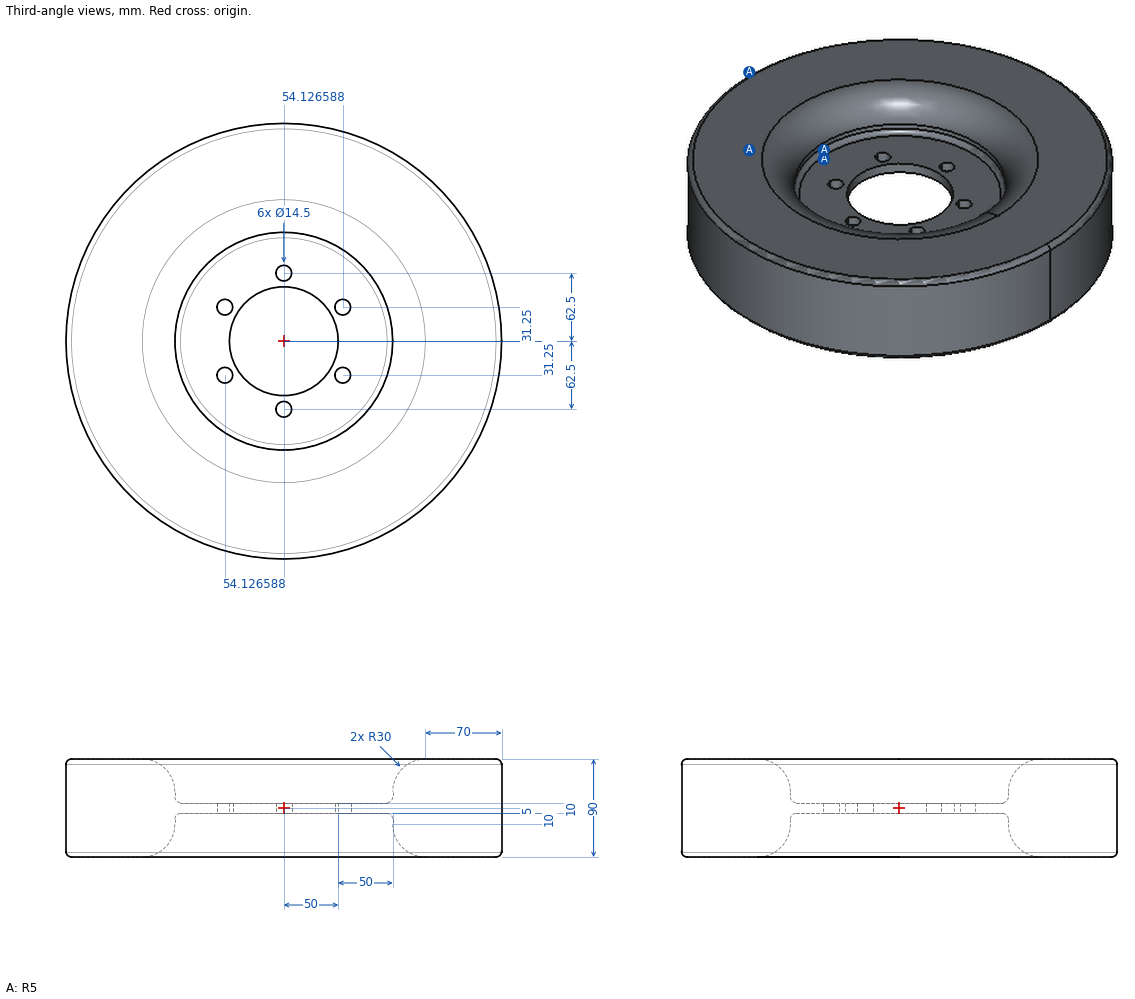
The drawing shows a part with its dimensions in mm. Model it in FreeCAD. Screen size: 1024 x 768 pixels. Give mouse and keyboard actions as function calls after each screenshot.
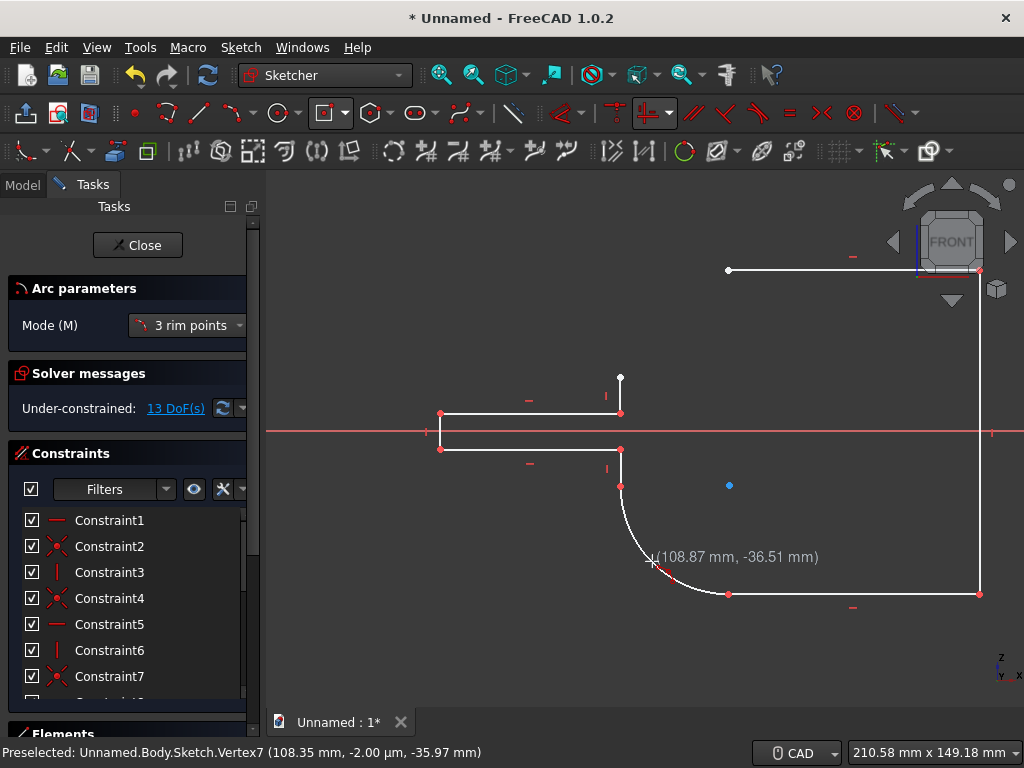
click(620, 378)
click(728, 270)
click(652, 300)
key(Escape)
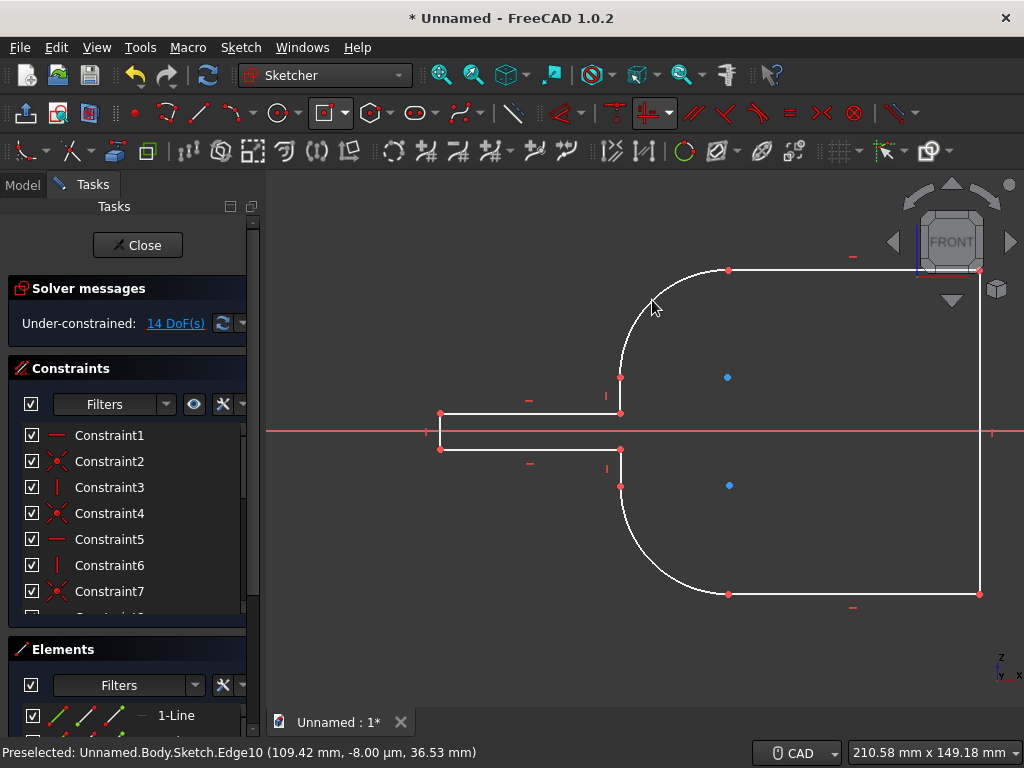
click(804, 270)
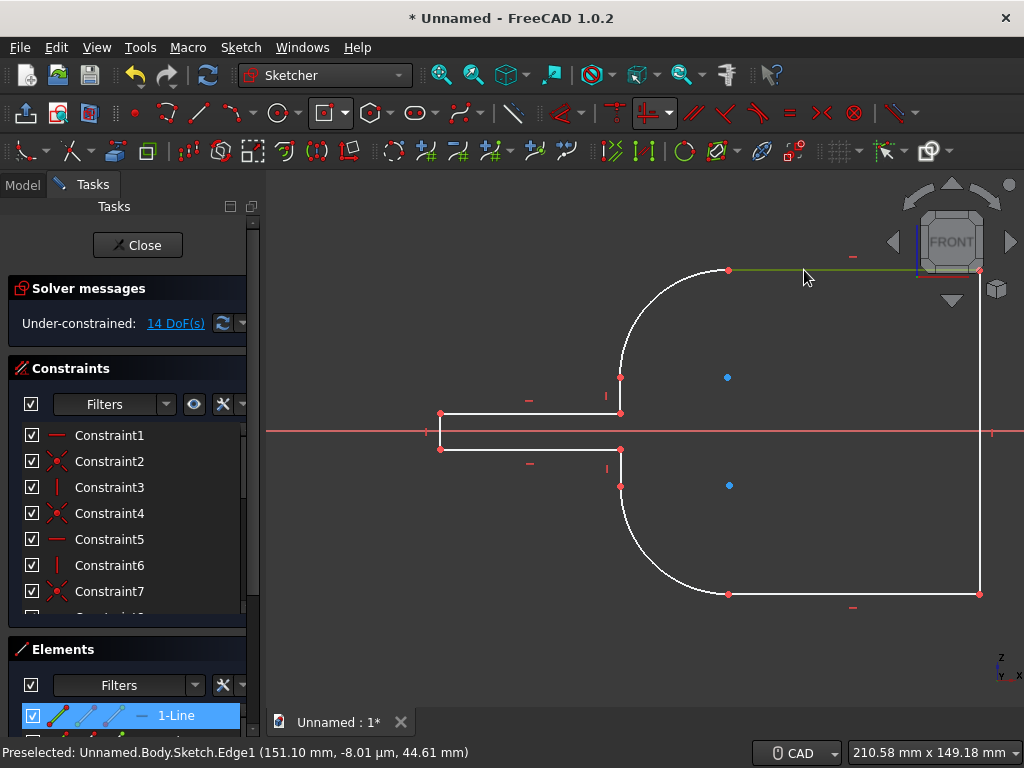
click(679, 282)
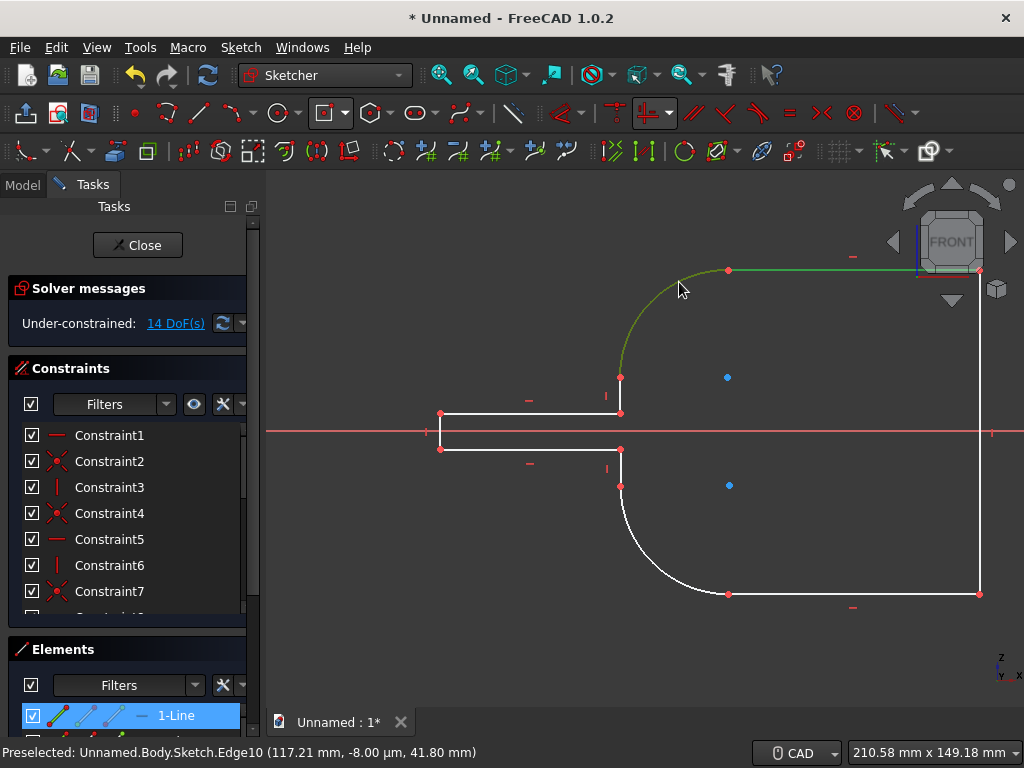
click(758, 114)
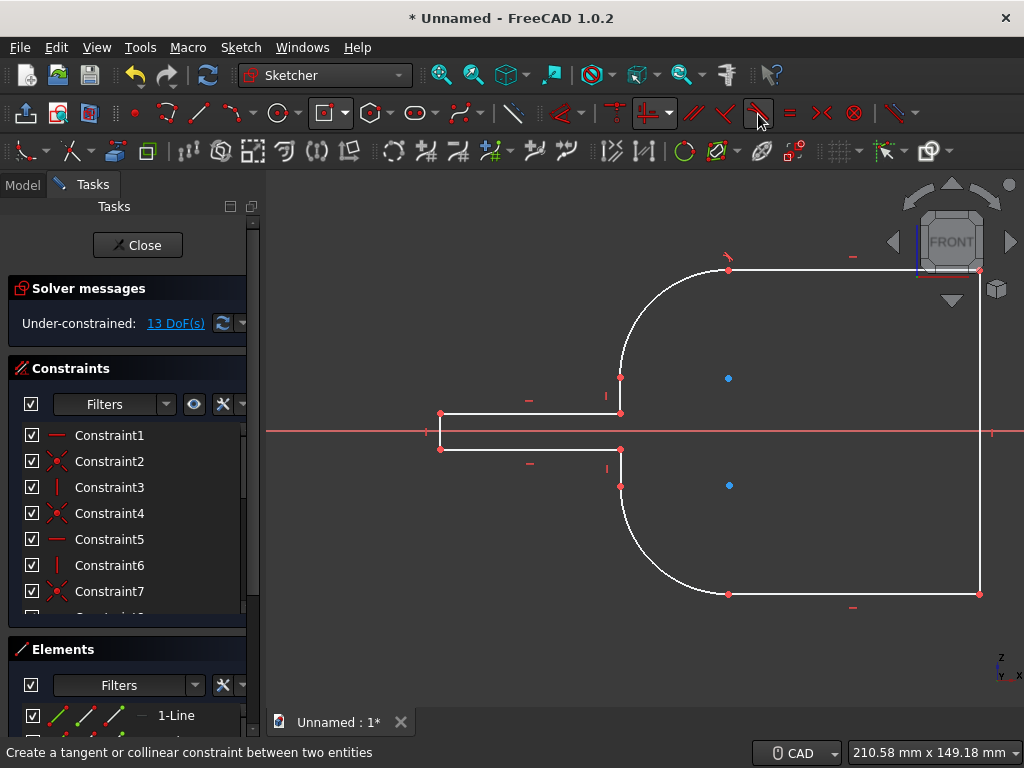
click(804, 594)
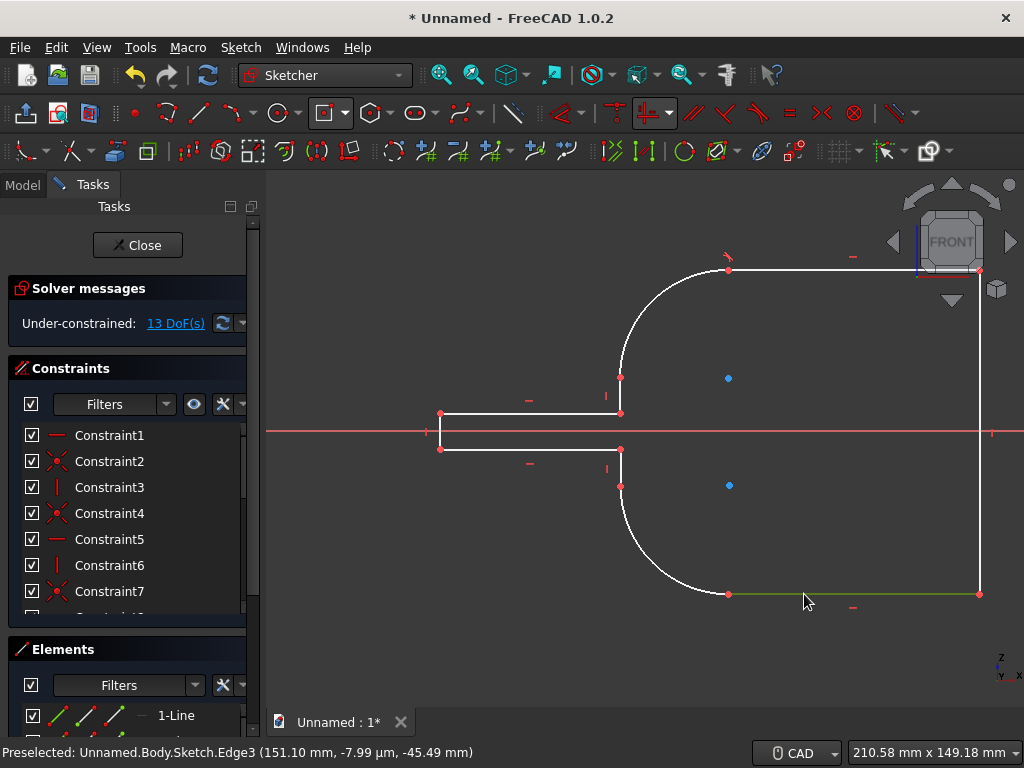
click(633, 535)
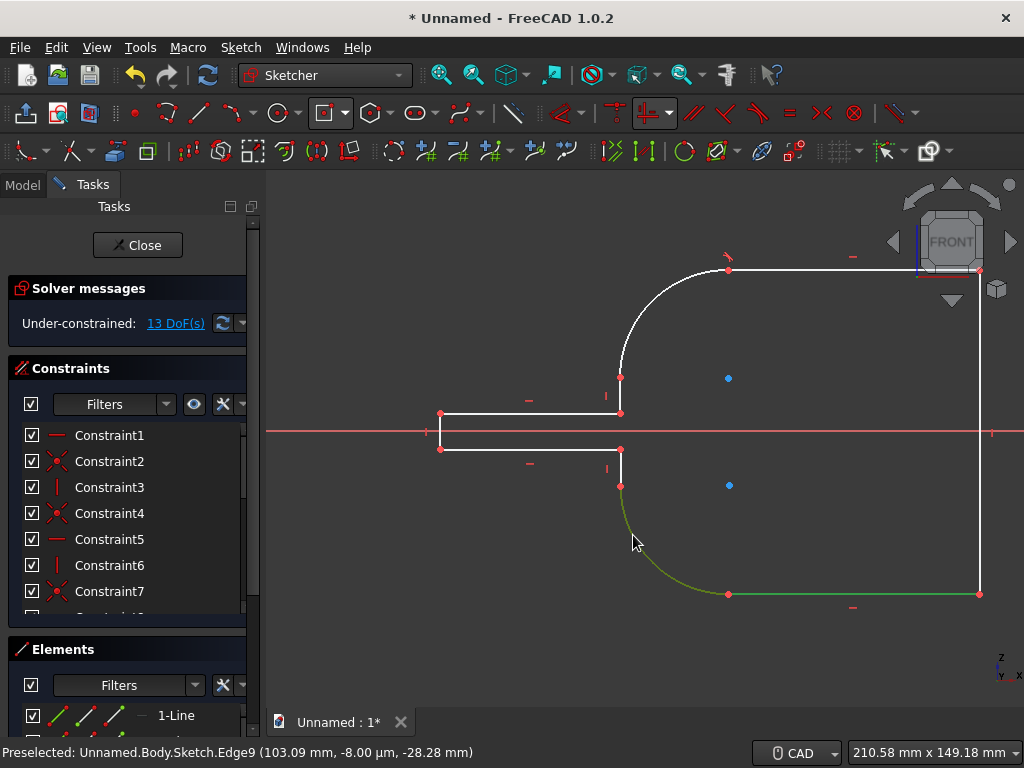
click(758, 114)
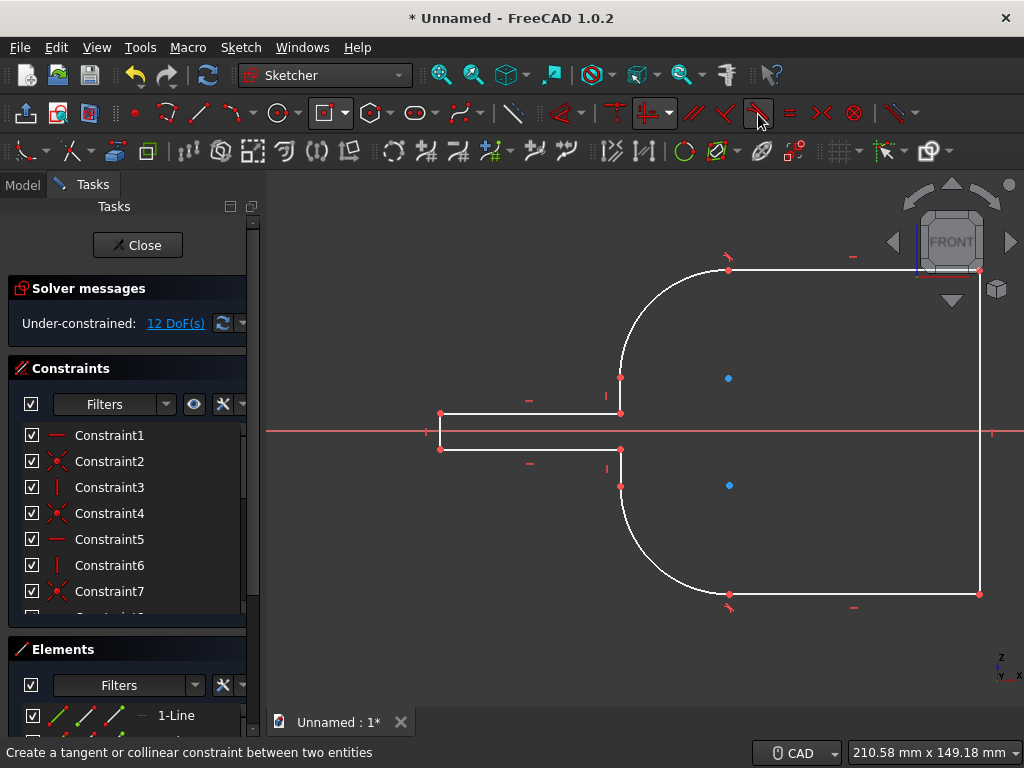
scroll(621, 476, up, 2)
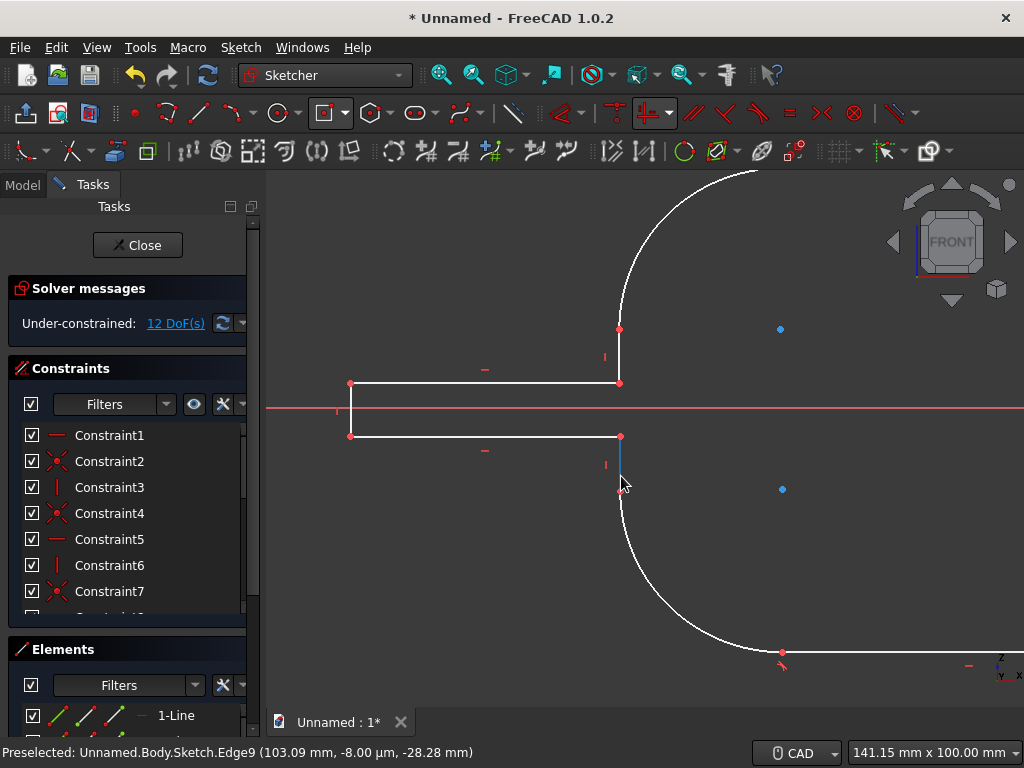
click(620, 475)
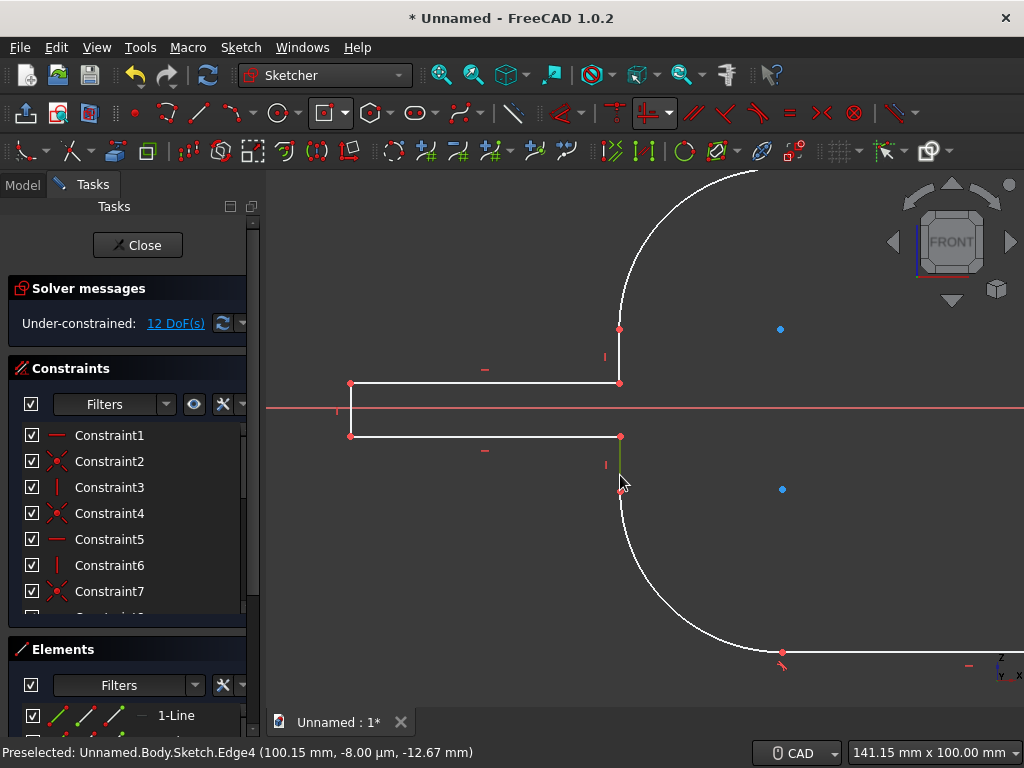
click(638, 565)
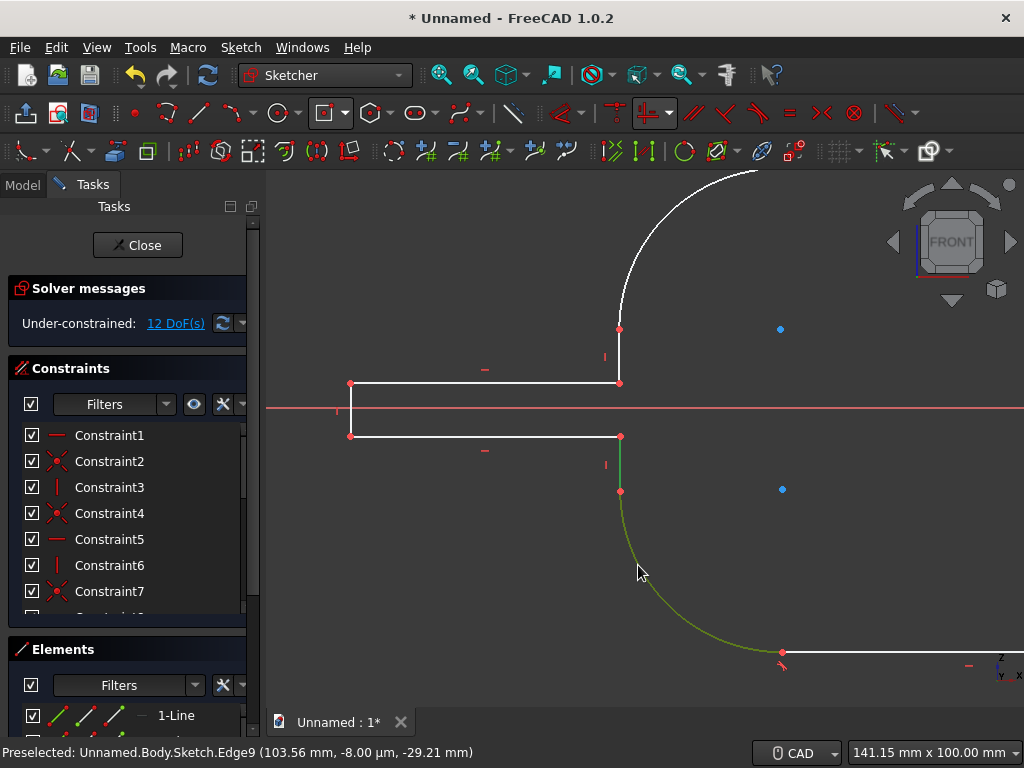
click(758, 114)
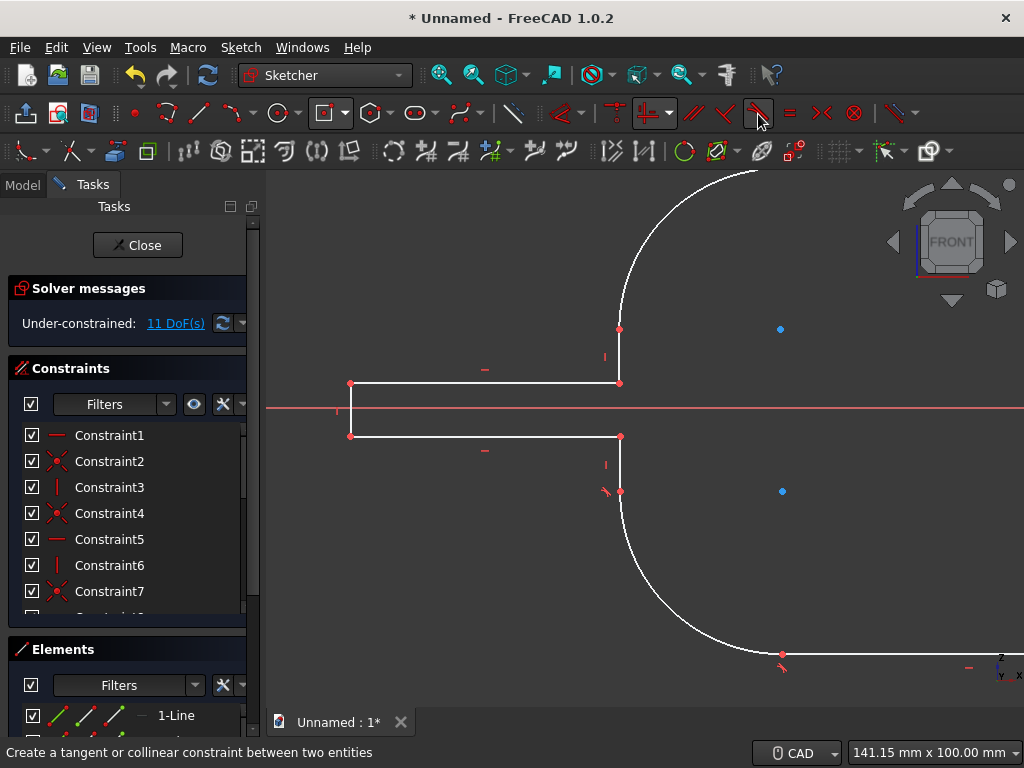
click(619, 367)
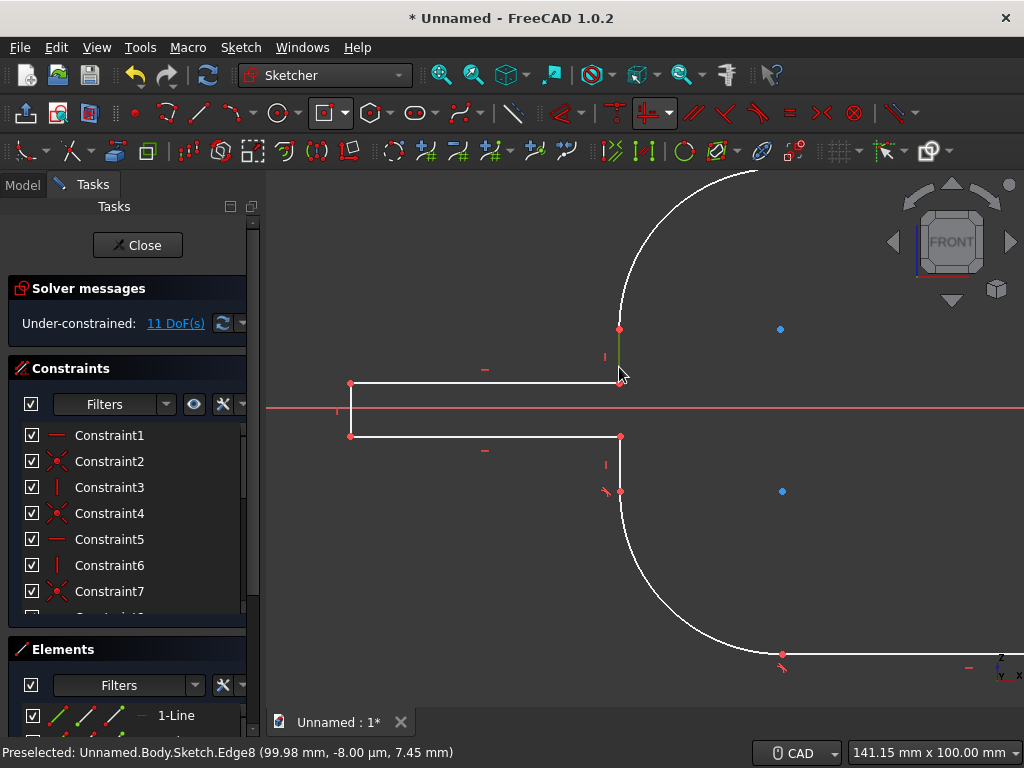
click(637, 256)